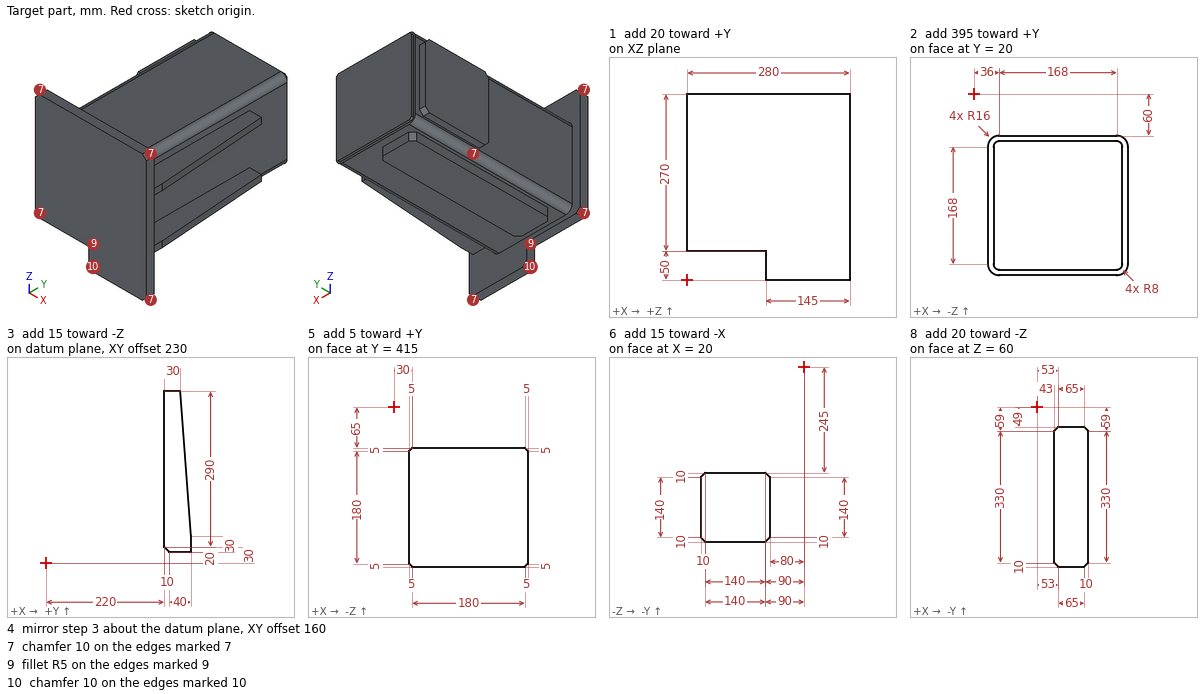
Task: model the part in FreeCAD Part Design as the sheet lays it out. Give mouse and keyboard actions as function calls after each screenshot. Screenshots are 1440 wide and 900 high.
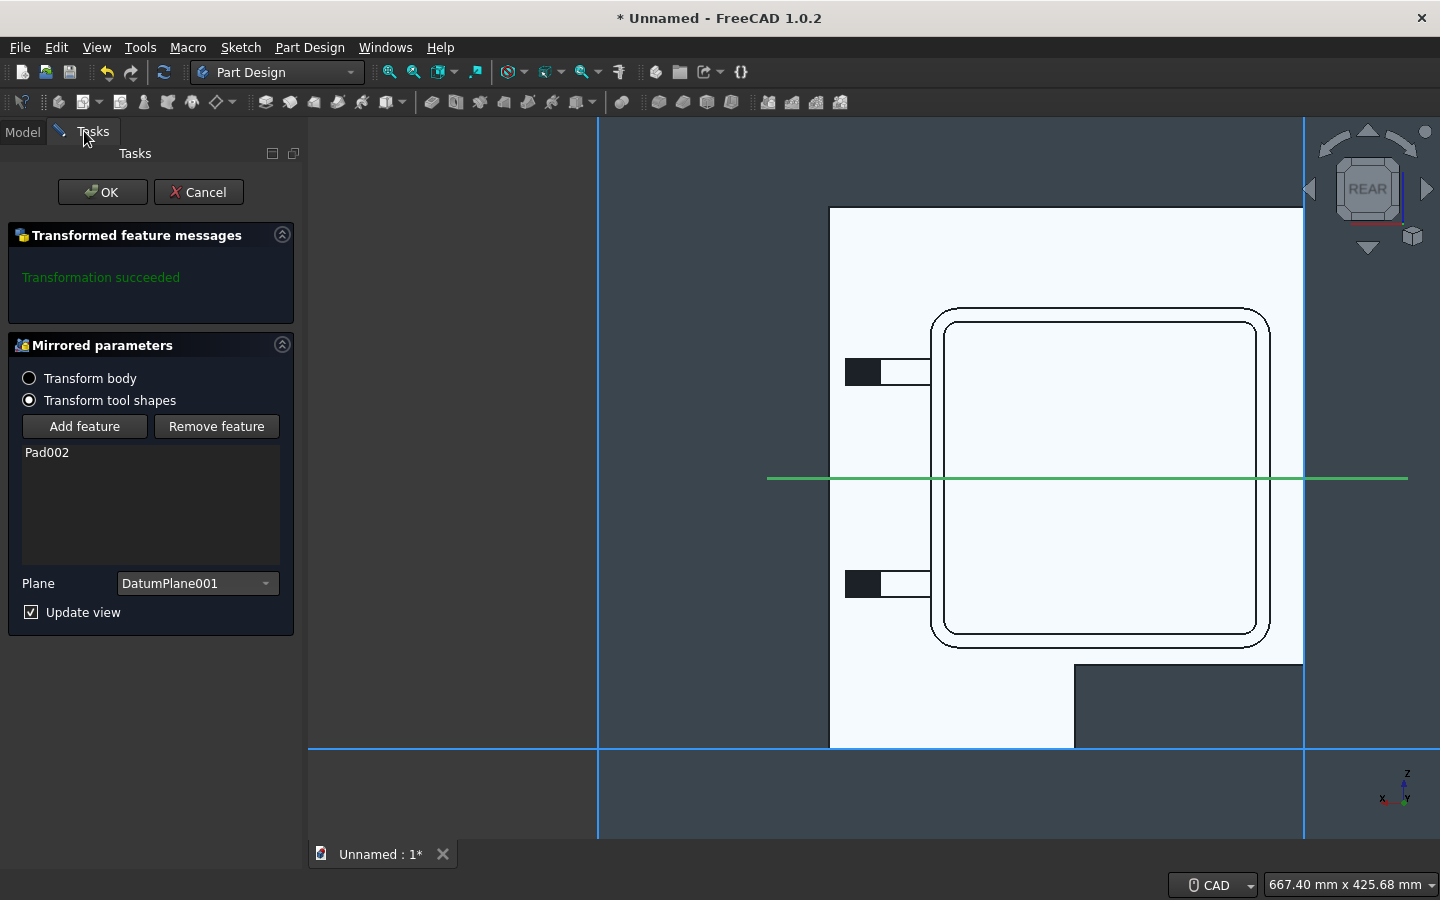
click(103, 192)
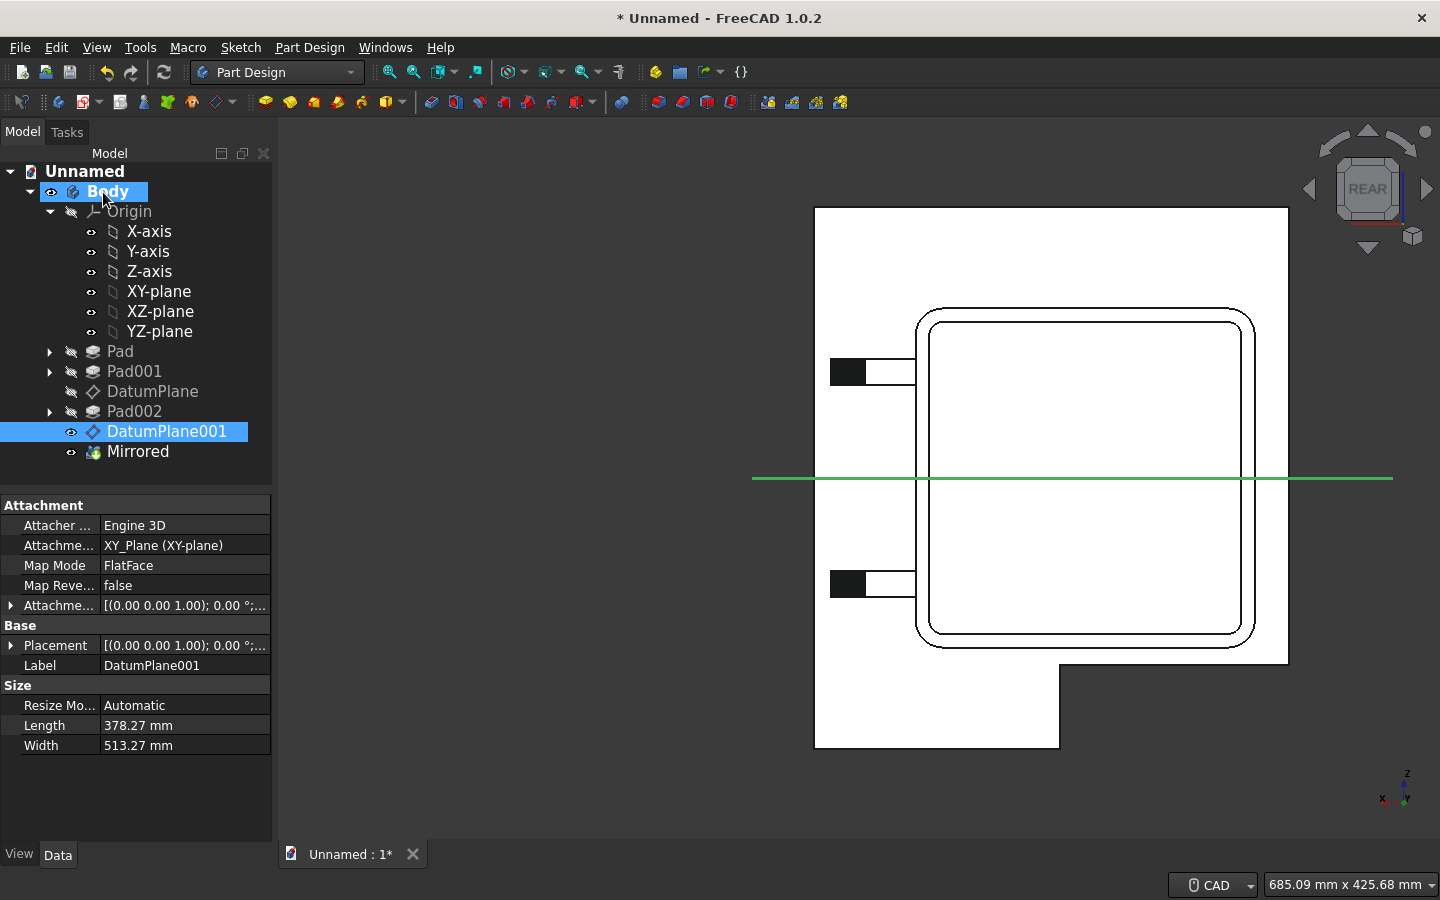
click(116, 432)
key(space)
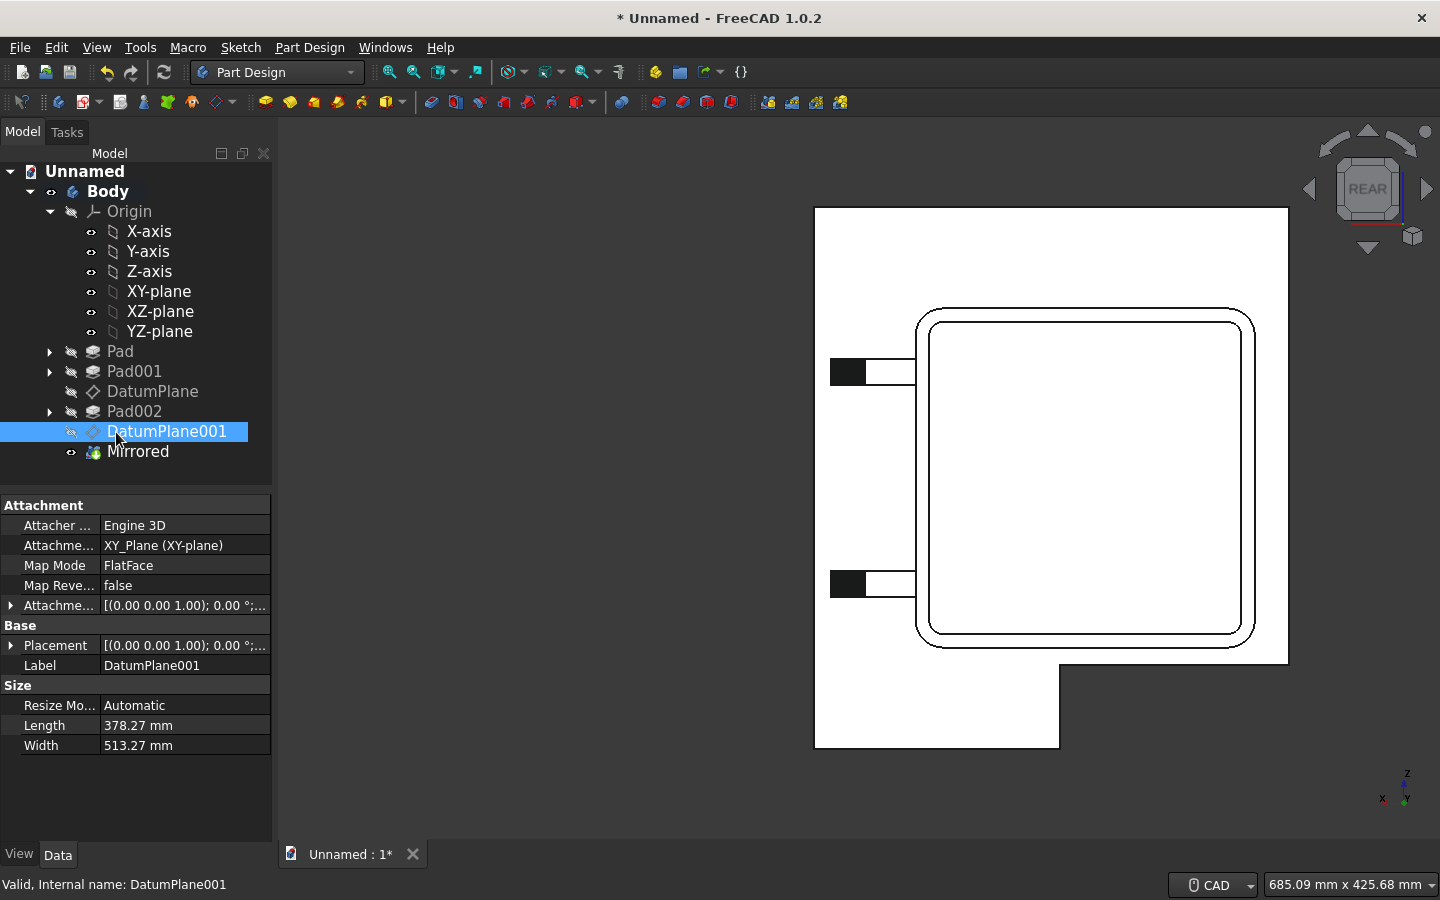
scroll(921, 328, up, 5)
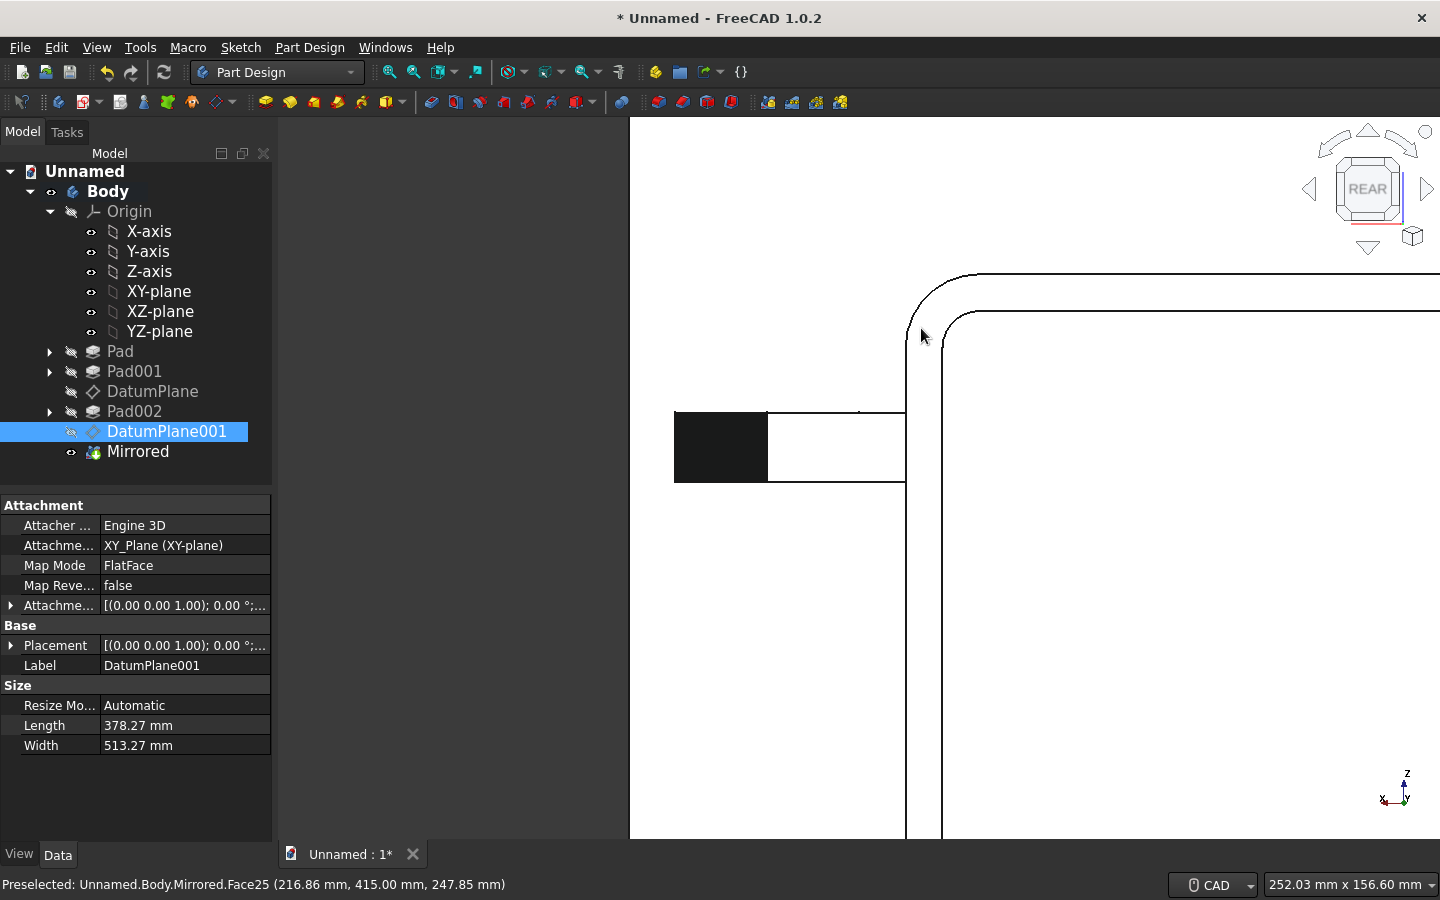
click(921, 328)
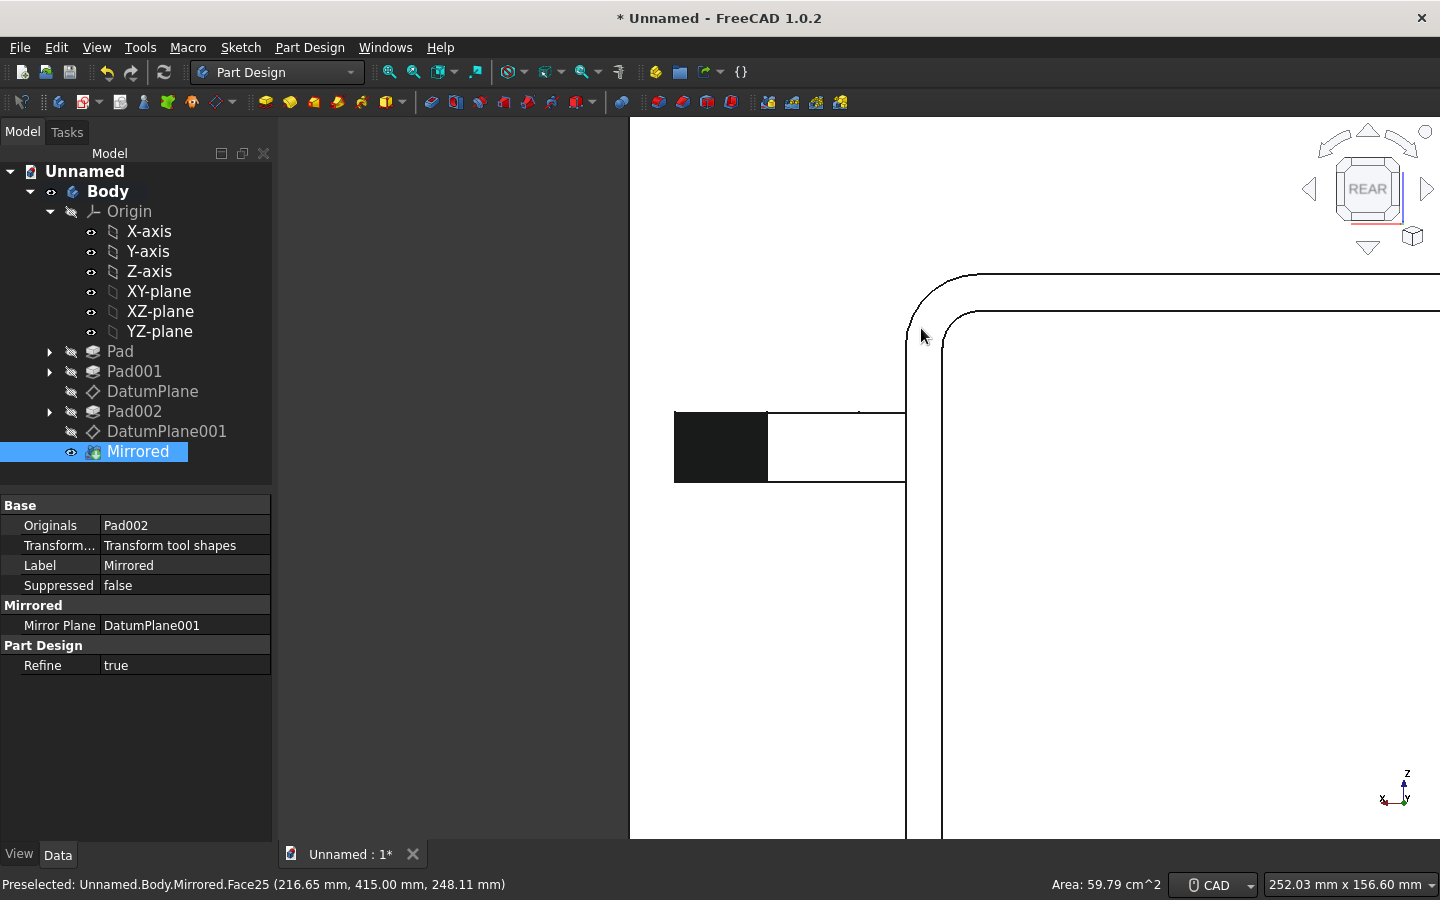
click(84, 102)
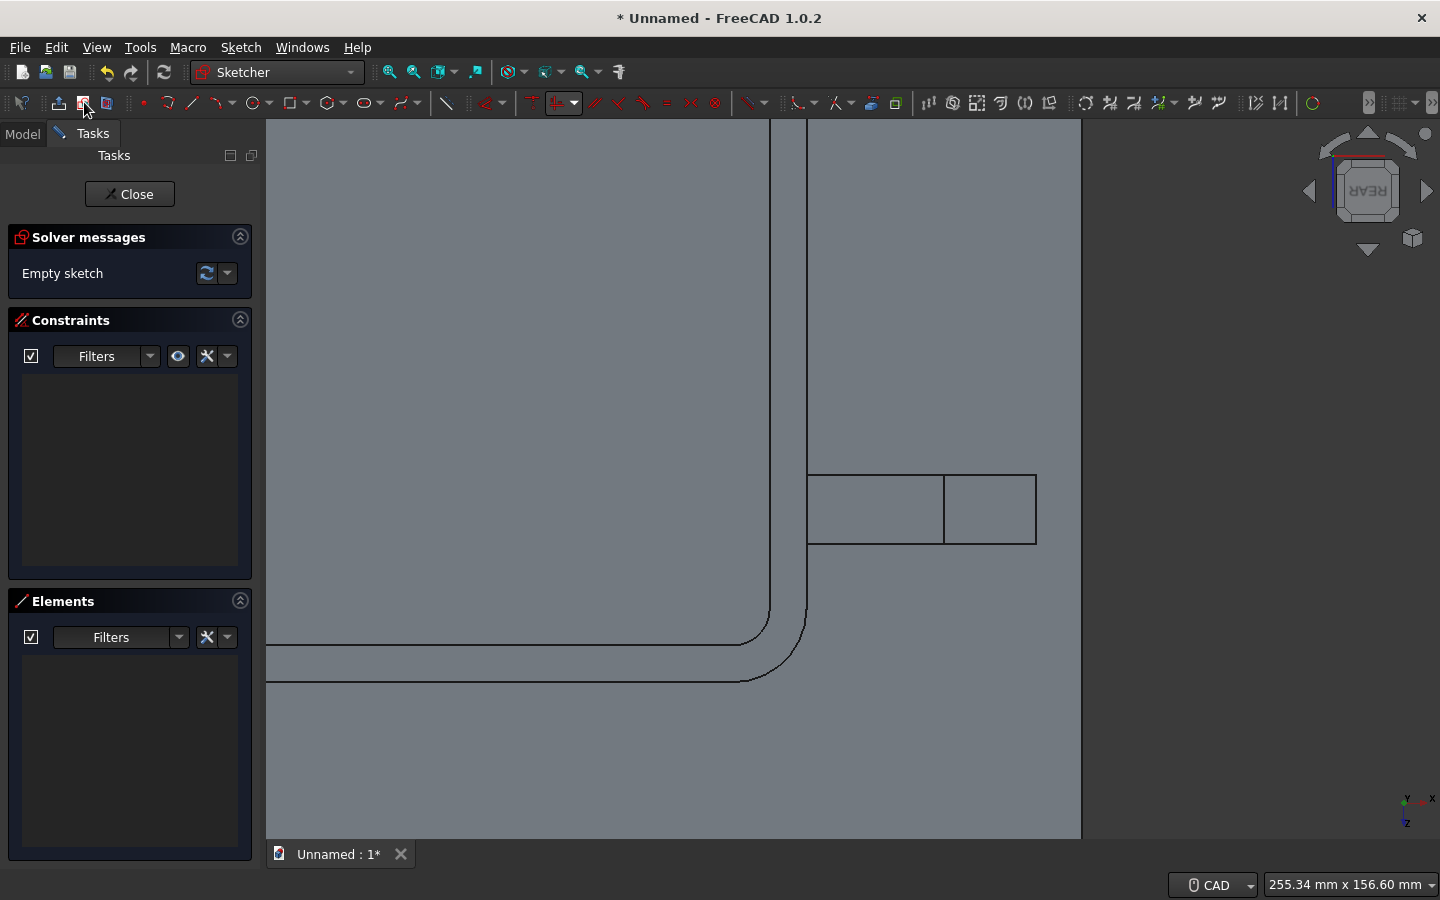
scroll(1073, 715, down, 5)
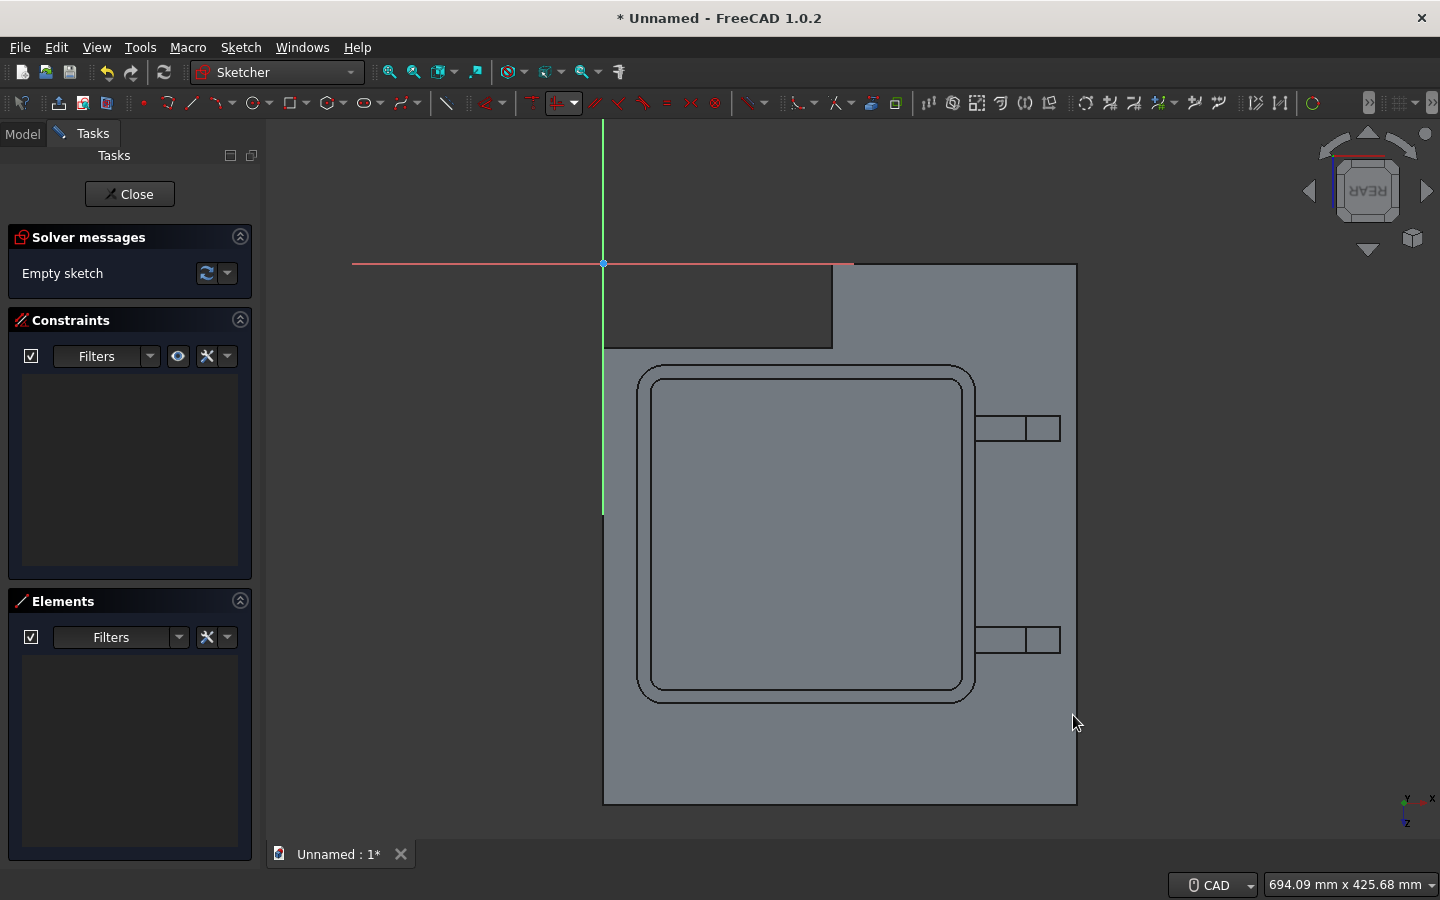
click(168, 104)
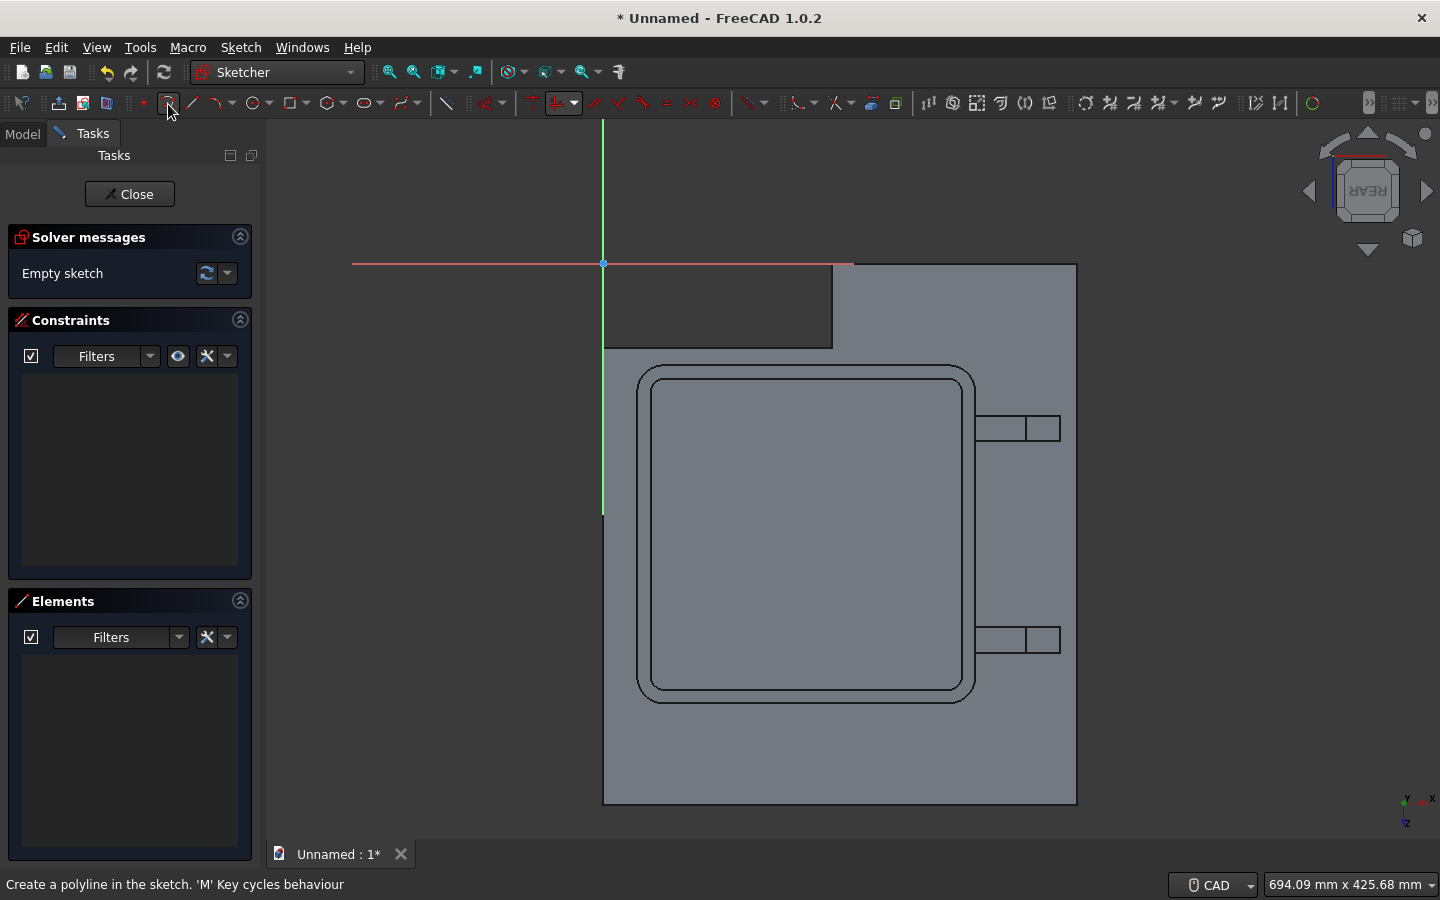
click(654, 374)